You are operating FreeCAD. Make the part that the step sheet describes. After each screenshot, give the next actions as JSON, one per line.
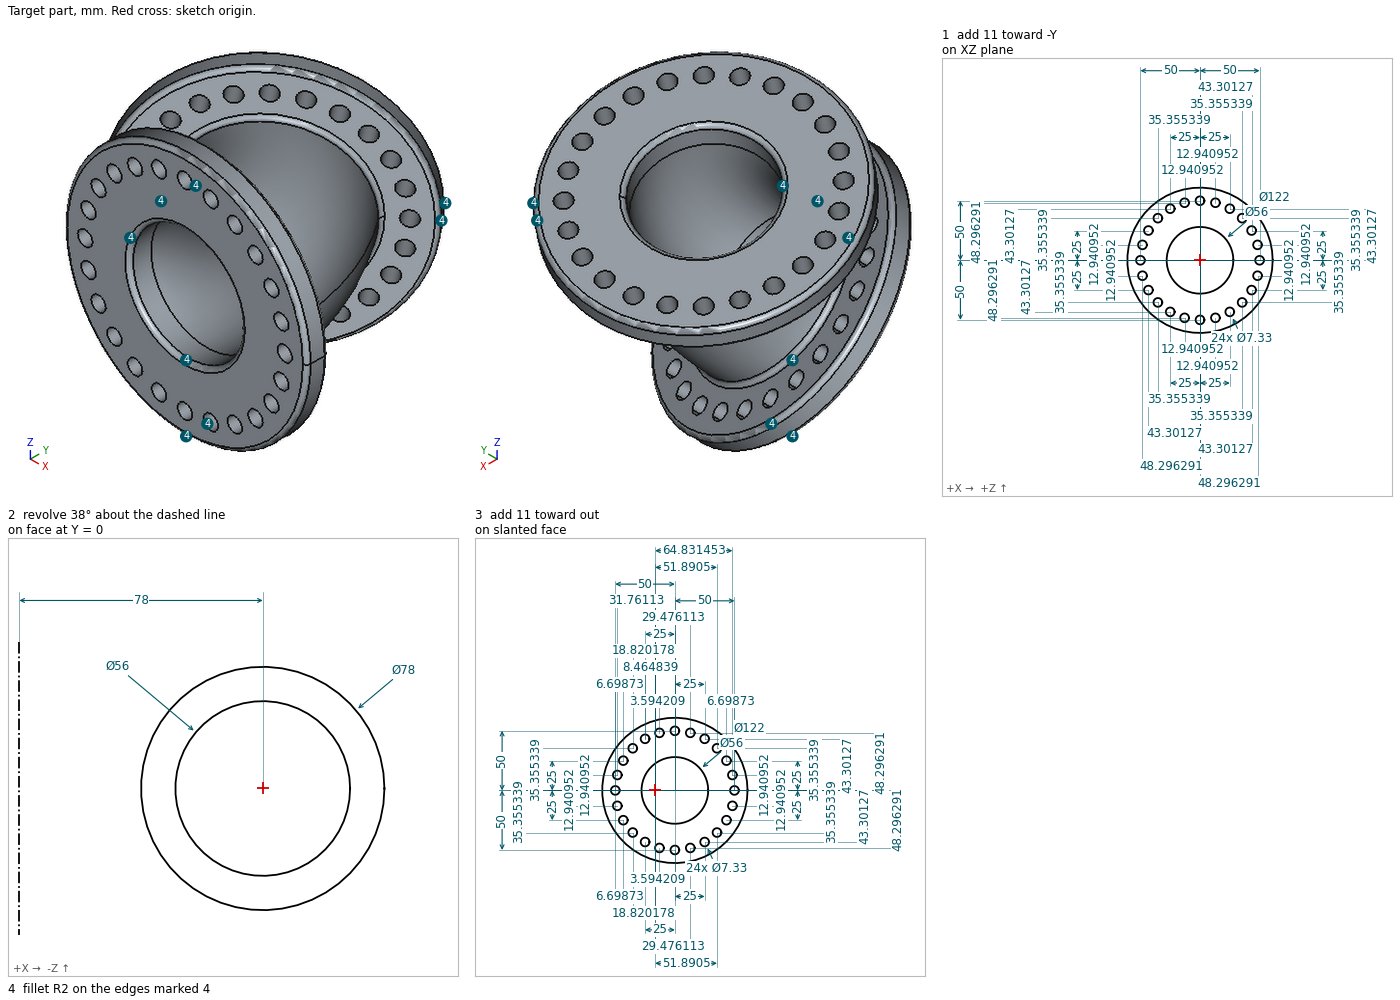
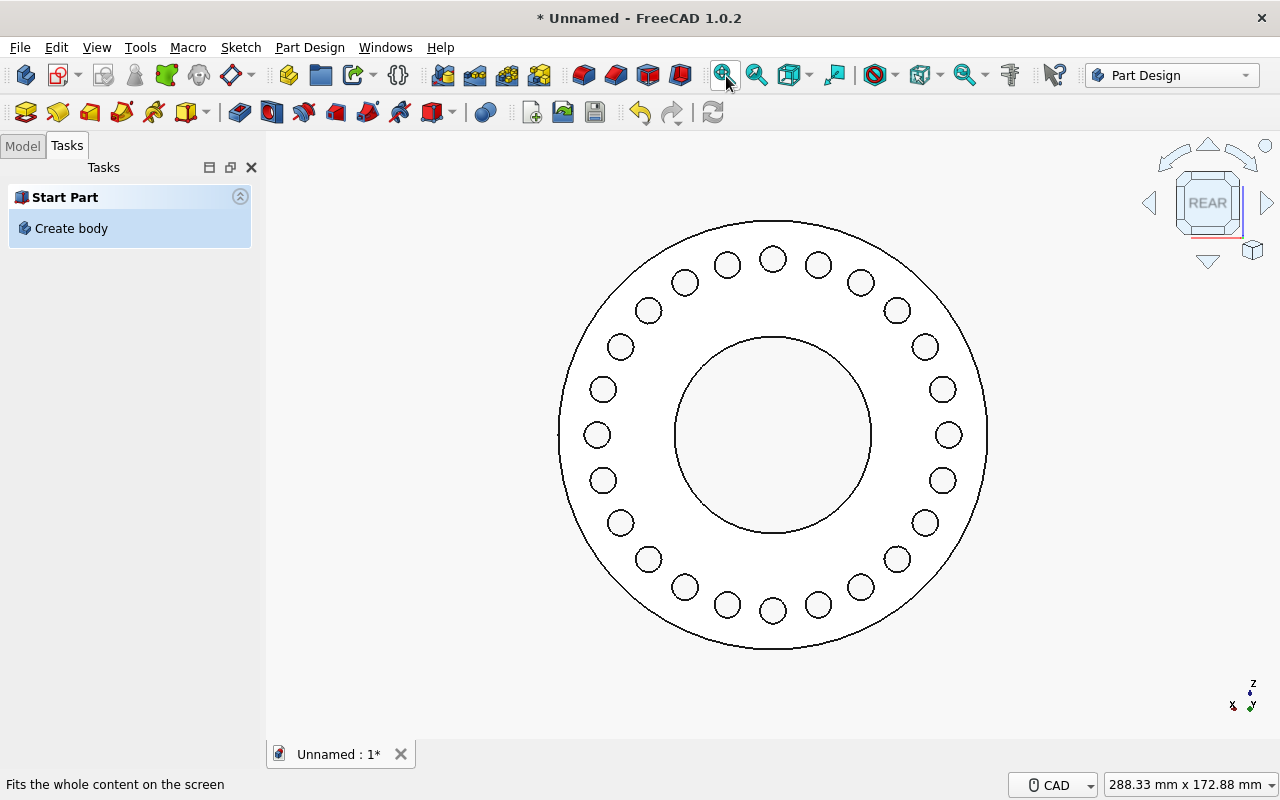
{"action": "left_click", "coordinate": [896, 373]}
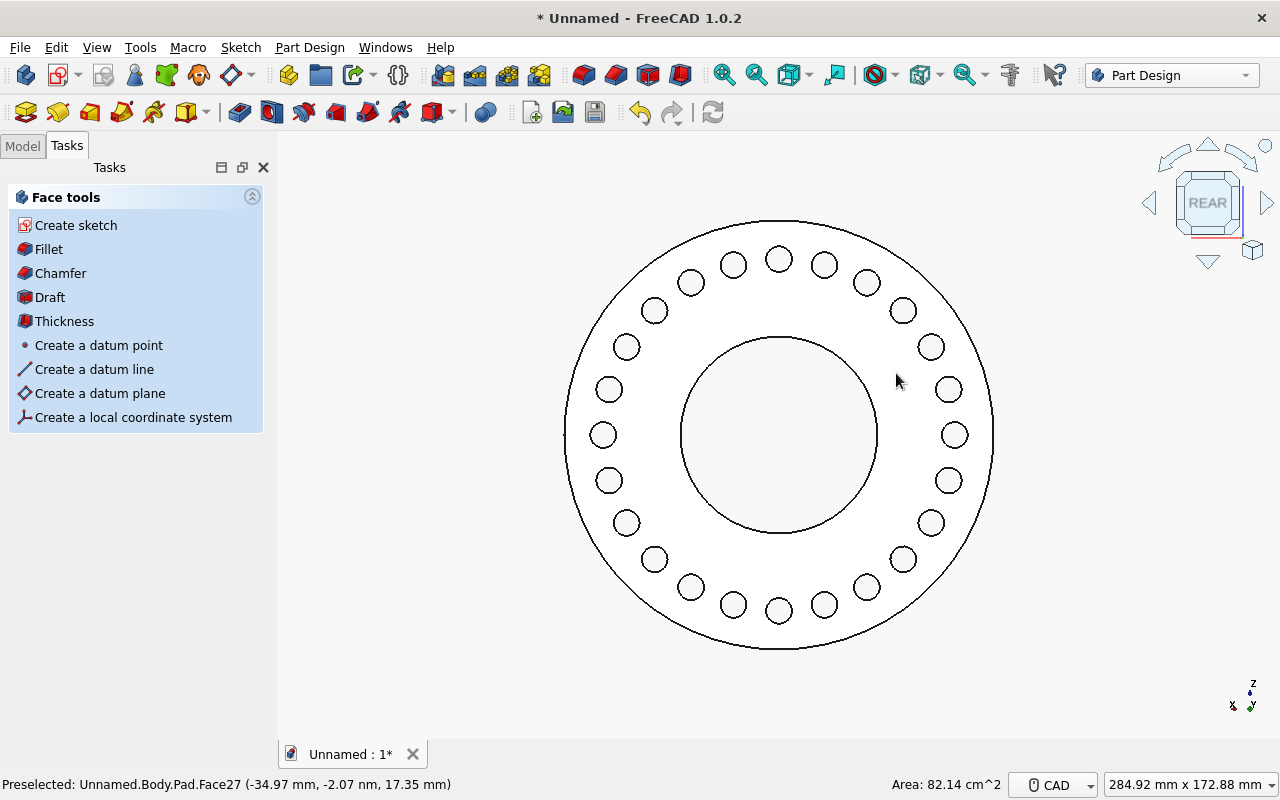
{"action": "left_click", "coordinate": [58, 76]}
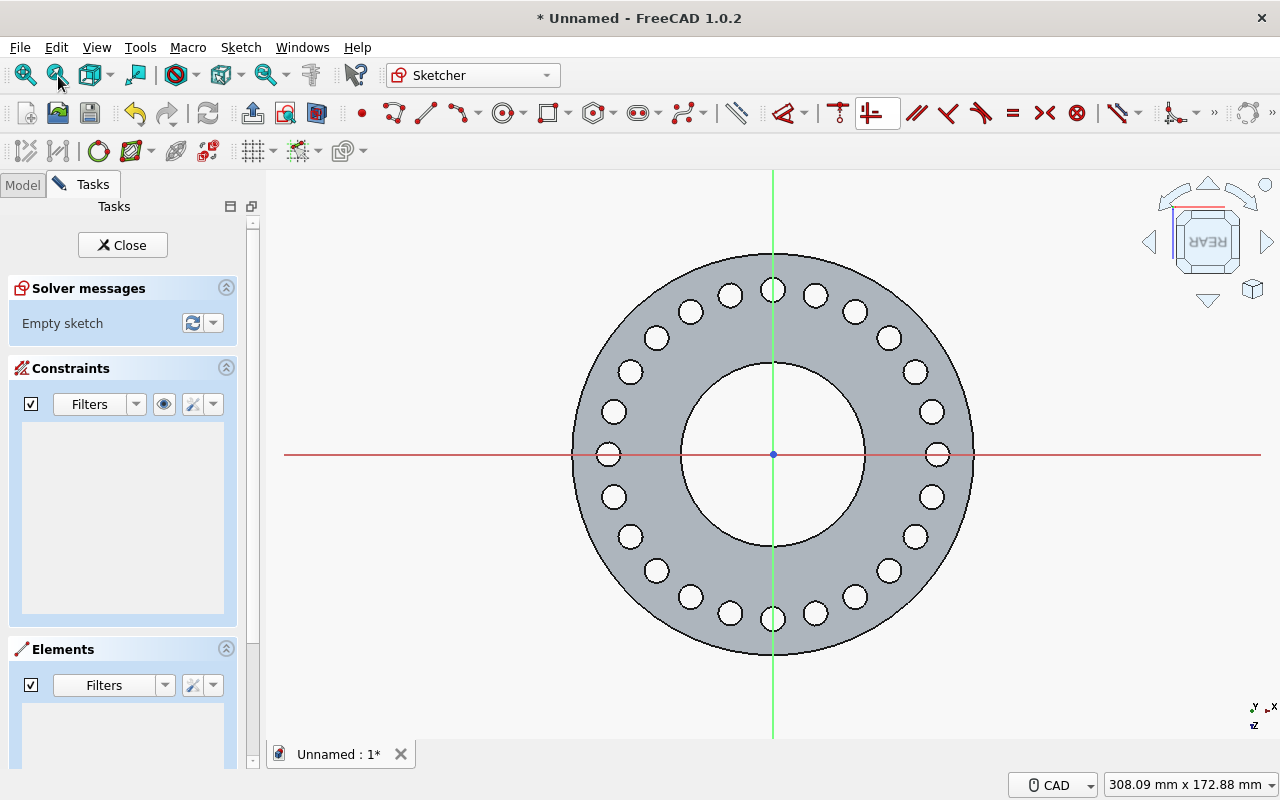
{"action": "left_click", "coordinate": [504, 114]}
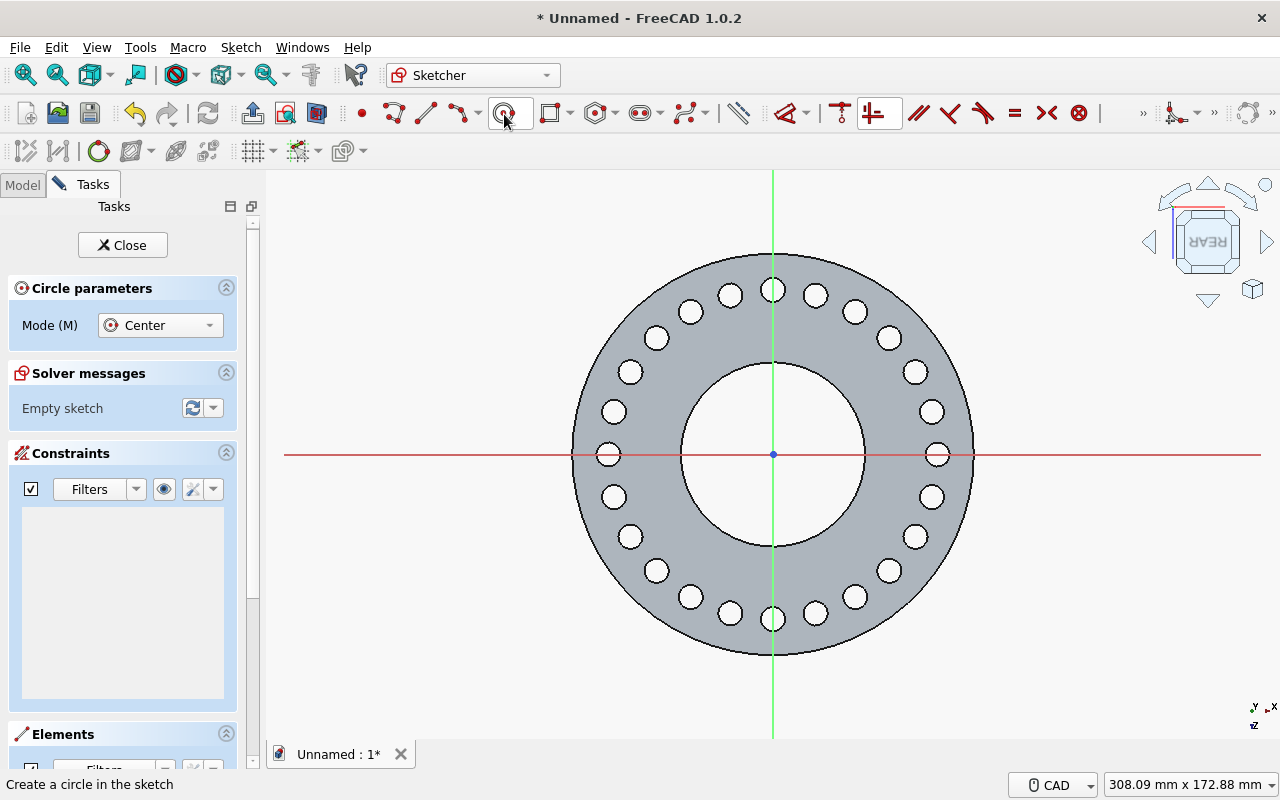
{"action": "left_click", "coordinate": [773, 455]}
{"action": "left_click", "coordinate": [864, 364]}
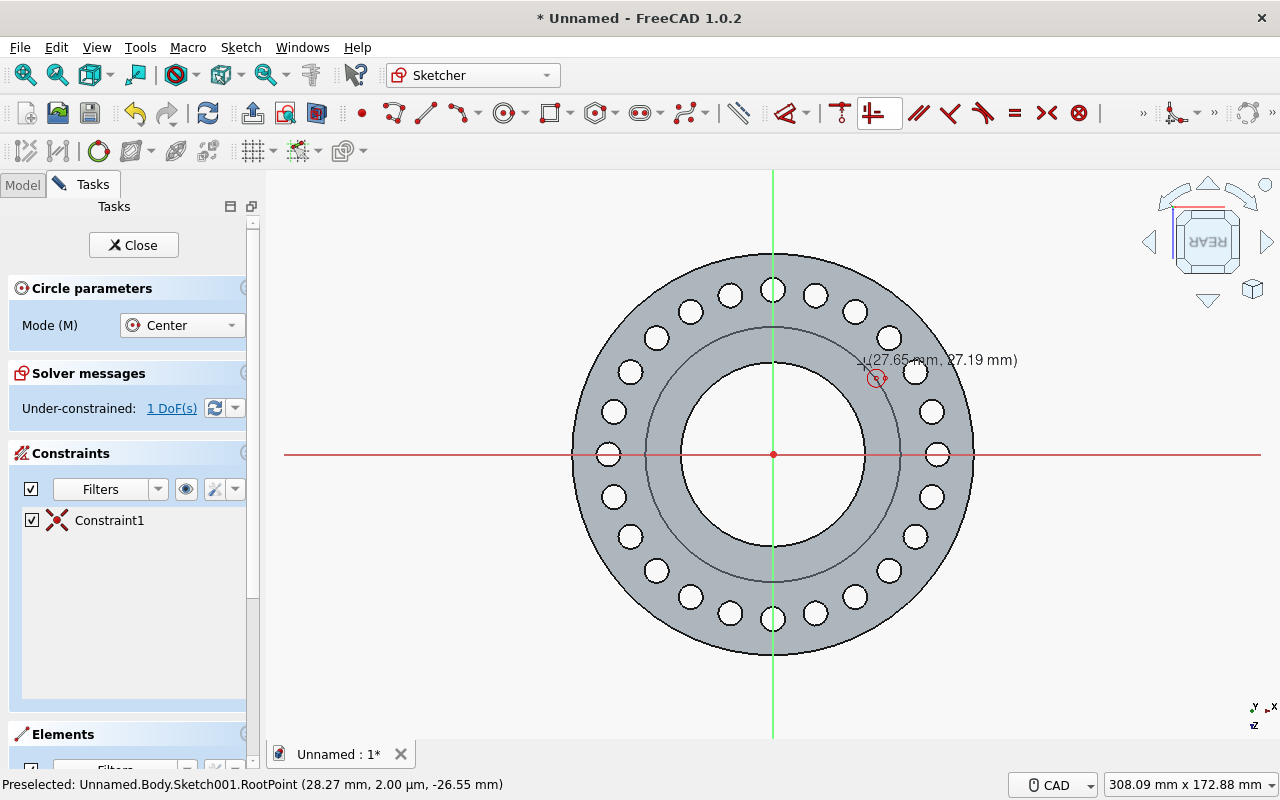
{"action": "left_click", "coordinate": [773, 455]}
{"action": "left_click", "coordinate": [838, 389]}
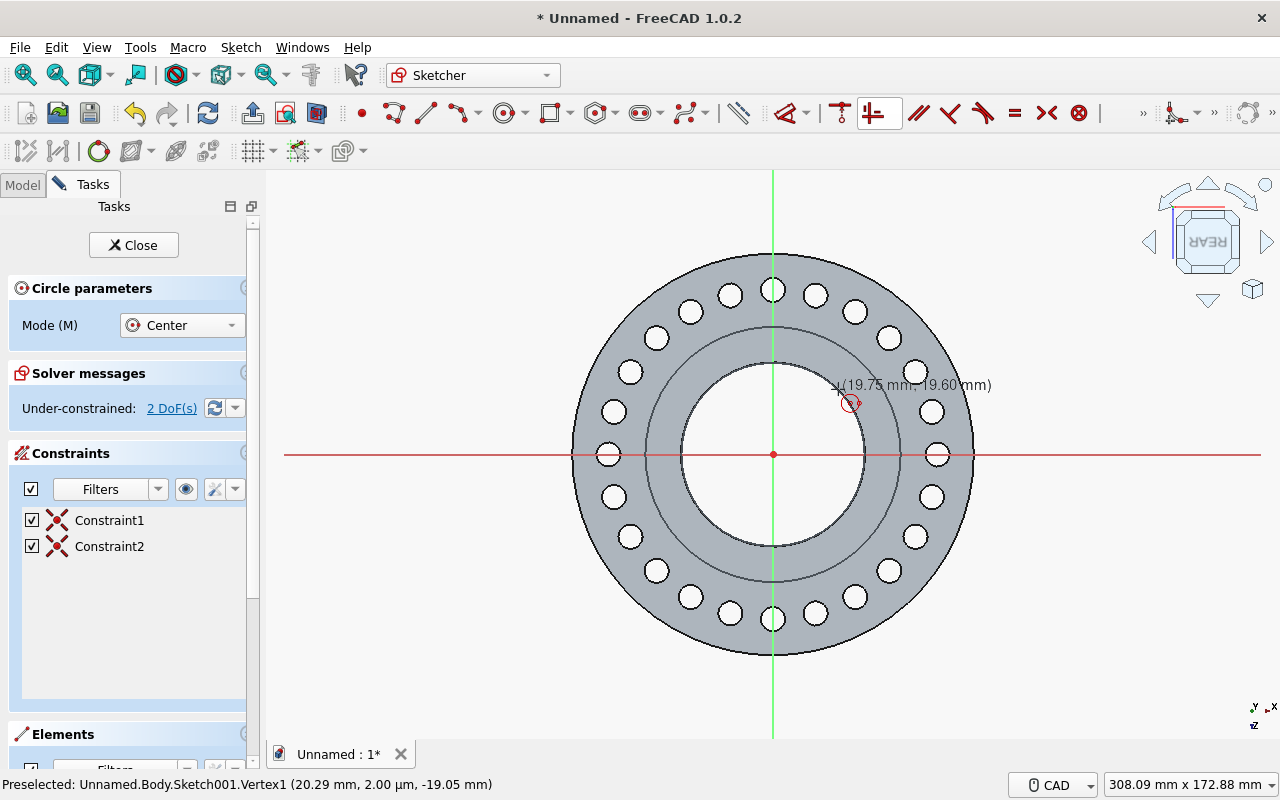
{"action": "left_click", "coordinate": [426, 114]}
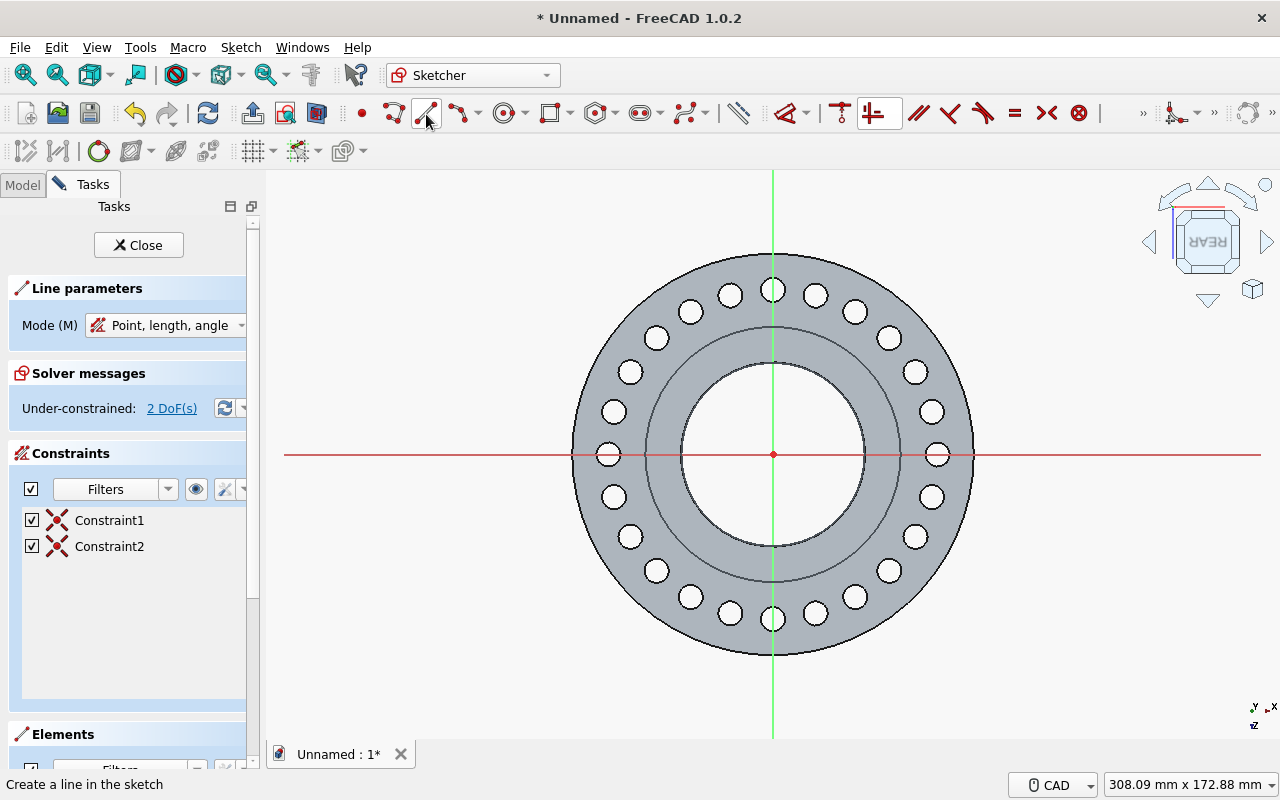
{"action": "left_click", "coordinate": [516, 300]}
{"action": "left_click", "coordinate": [516, 609]}
{"action": "key", "text": "Escape"}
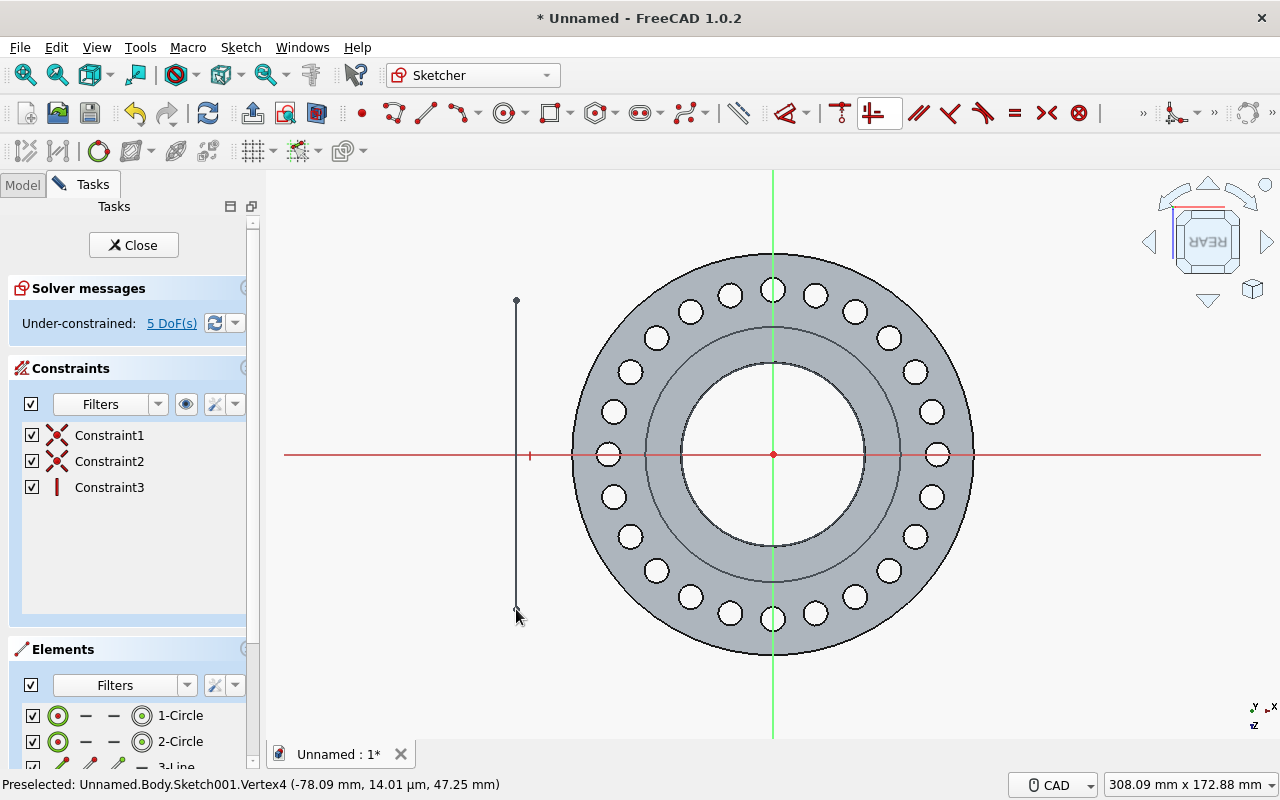
{"action": "left_click", "coordinate": [516, 394]}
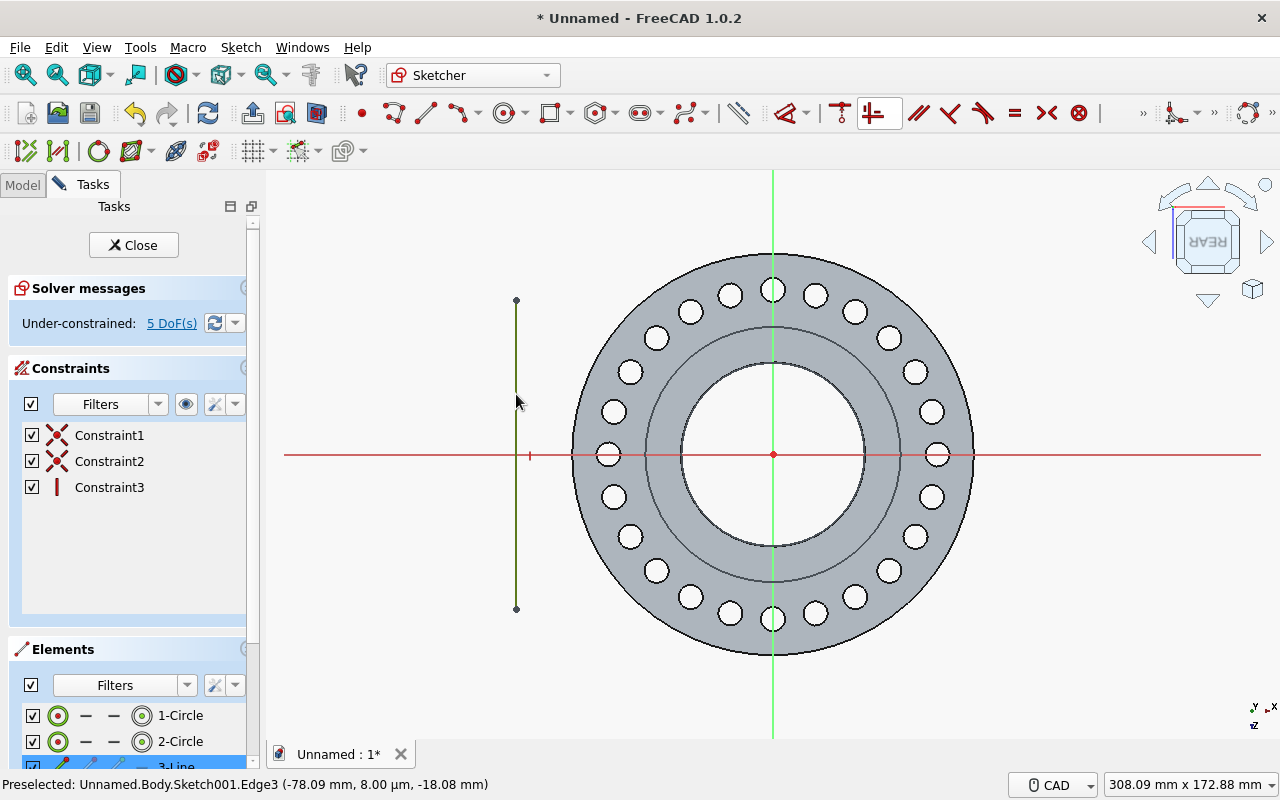
{"action": "left_click", "coordinate": [740, 114]}